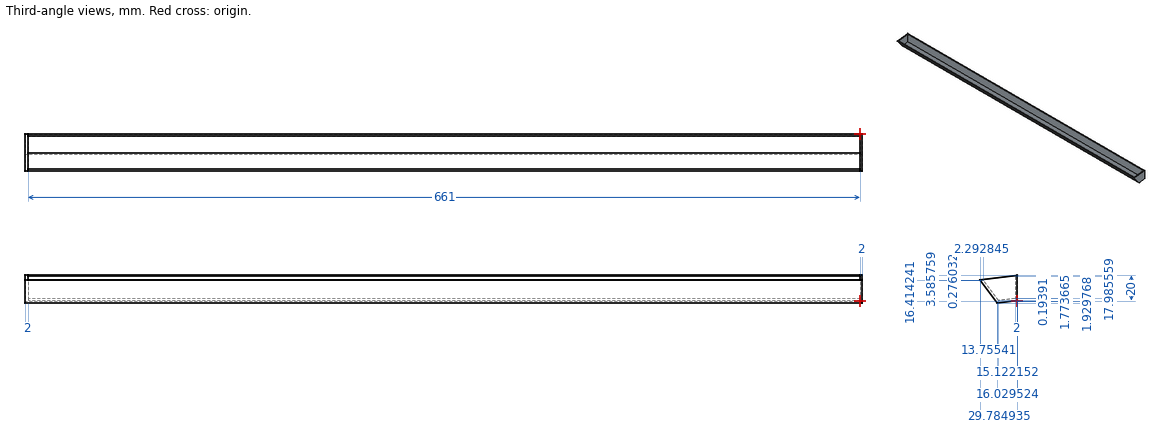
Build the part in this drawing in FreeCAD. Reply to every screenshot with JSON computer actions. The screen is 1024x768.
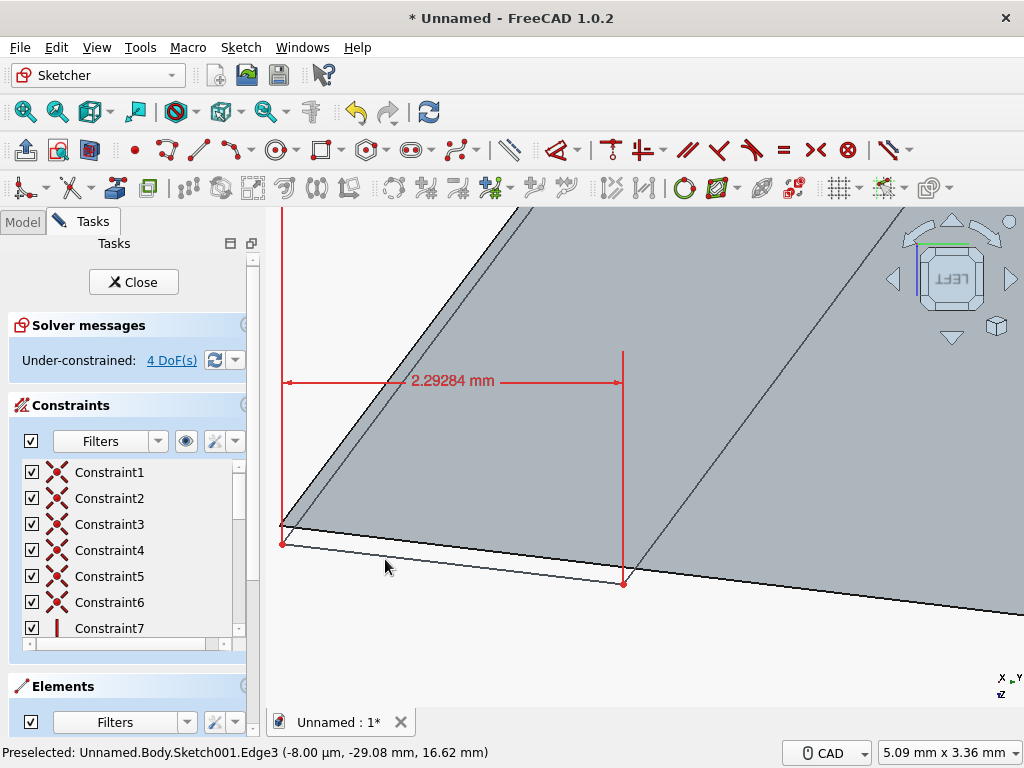
{"action": "left_click", "coordinate": [385, 556]}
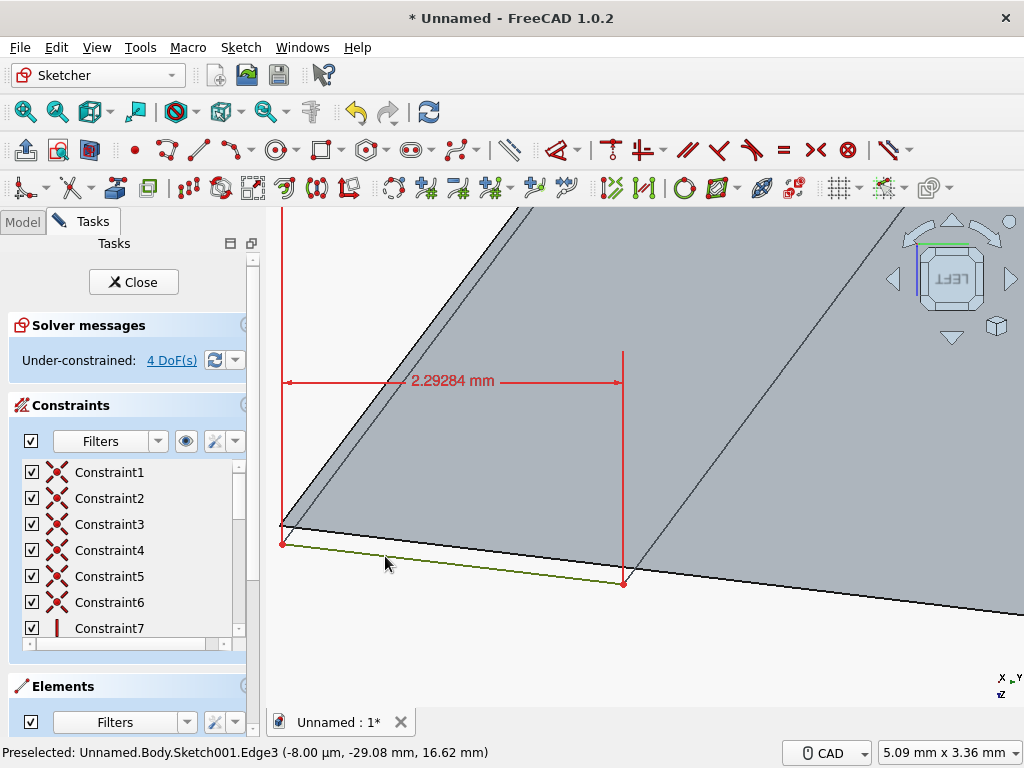
{"action": "left_click", "coordinate": [580, 150]}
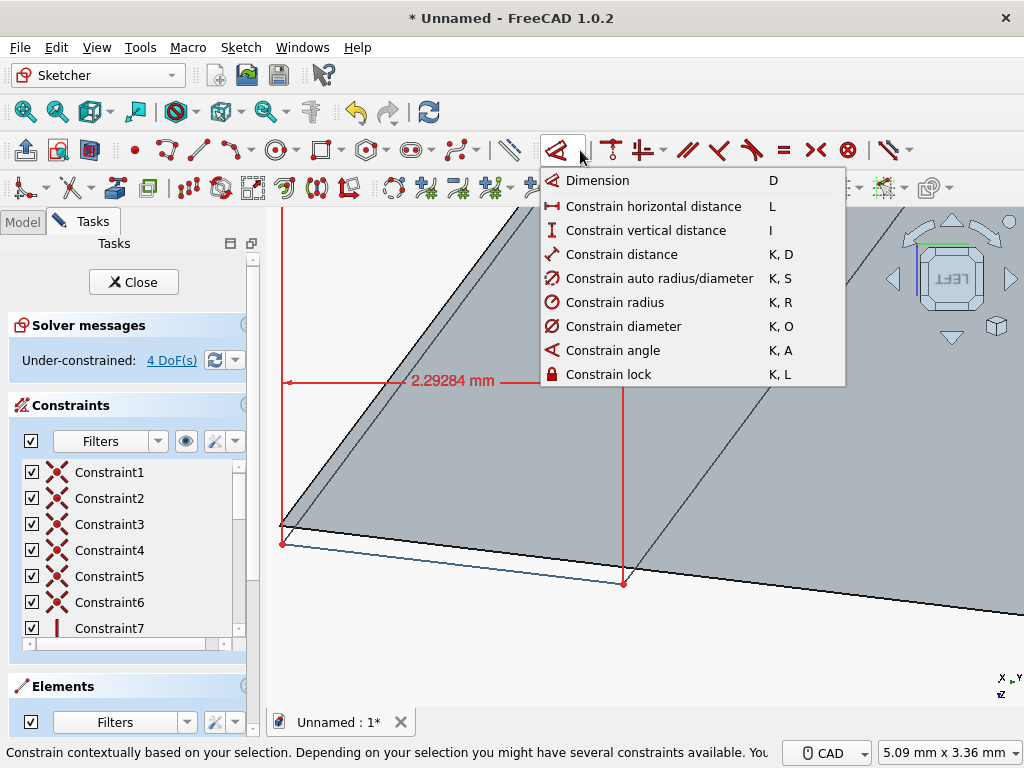
{"action": "left_click", "coordinate": [693, 230]}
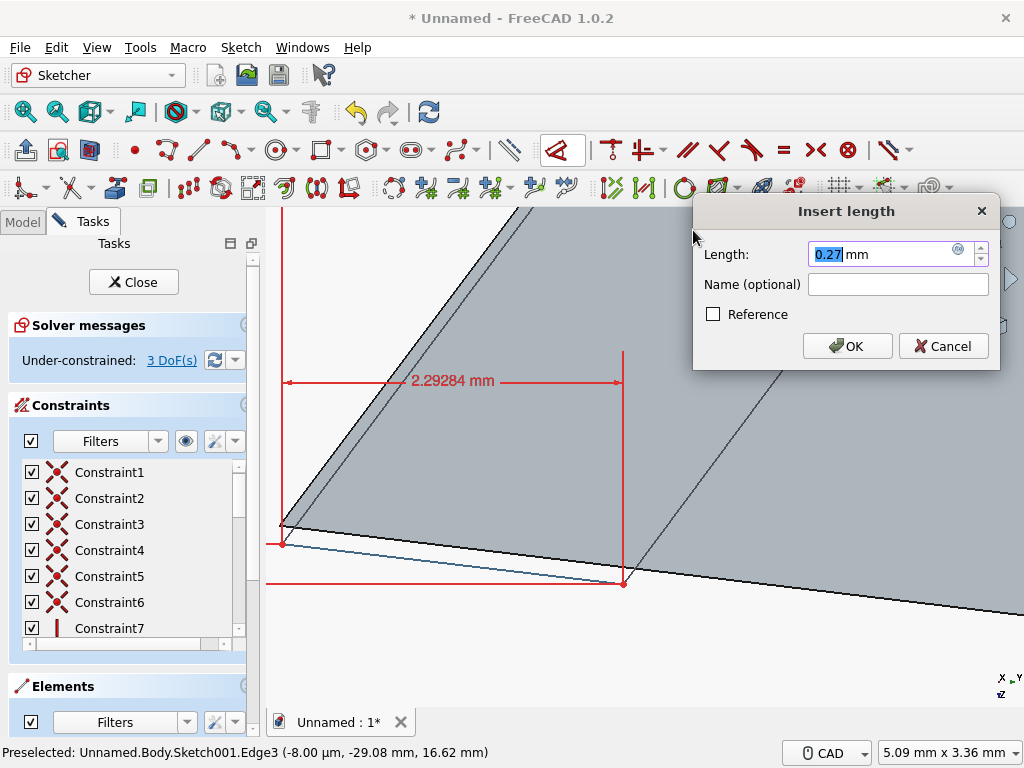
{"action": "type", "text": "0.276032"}
{"action": "key", "text": "Return"}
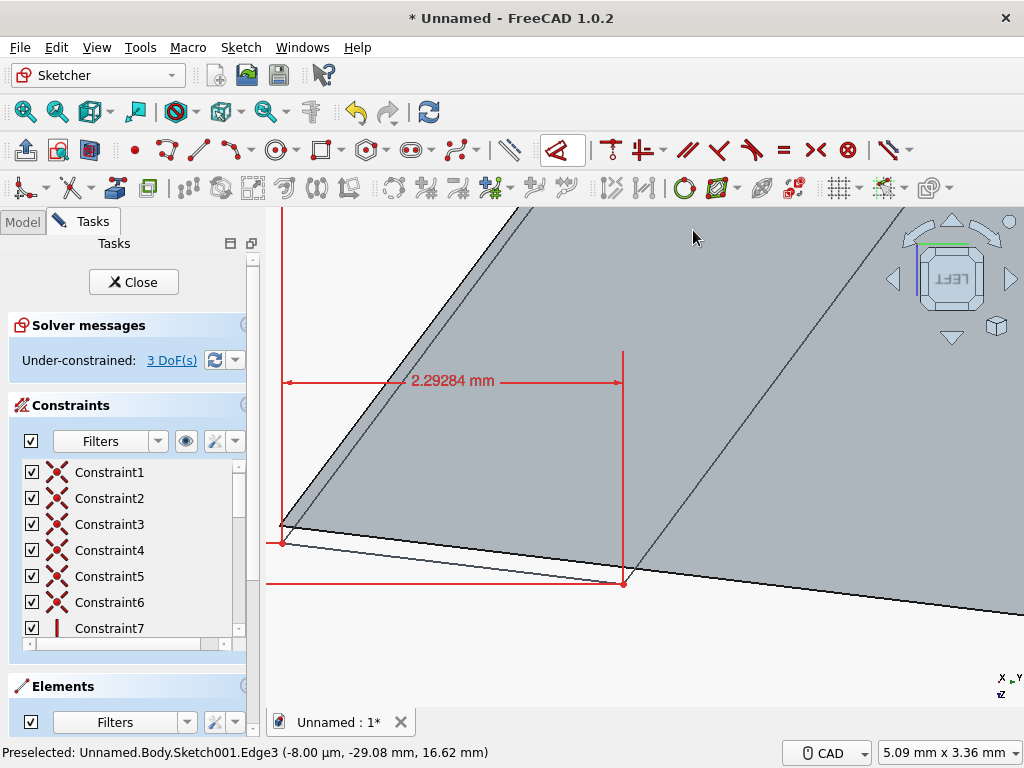
{"action": "scroll", "coordinate": [385, 560], "scroll_direction": "down", "scroll_amount": 12}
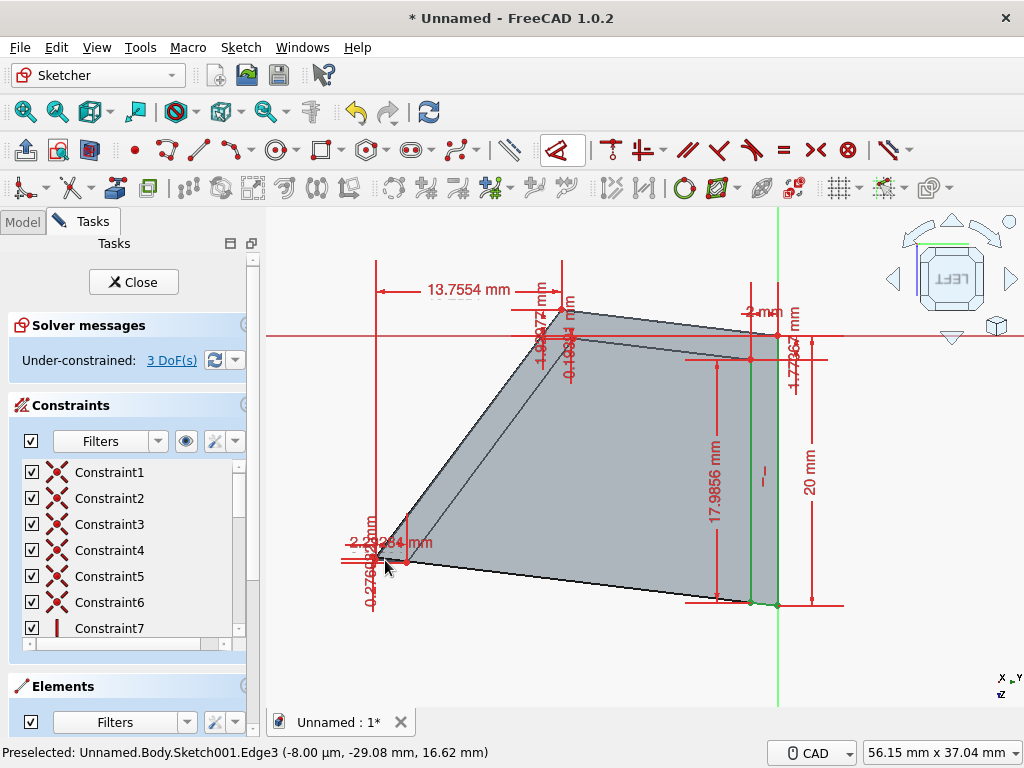
{"action": "left_click", "coordinate": [562, 310]}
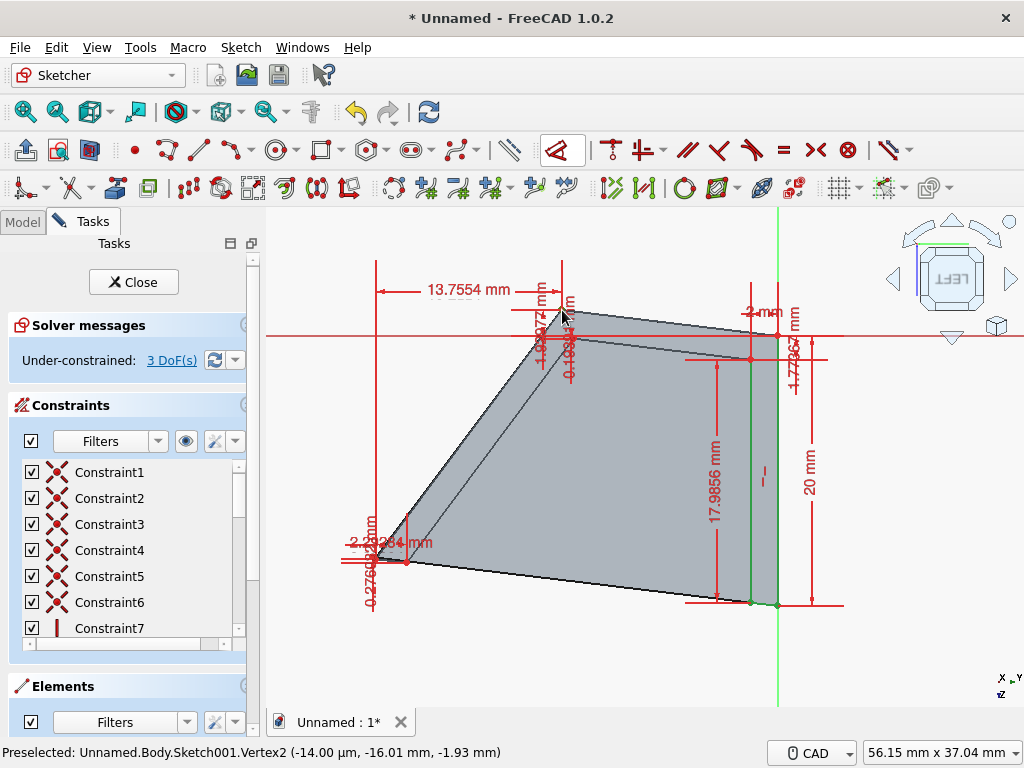
{"action": "key", "text": "l"}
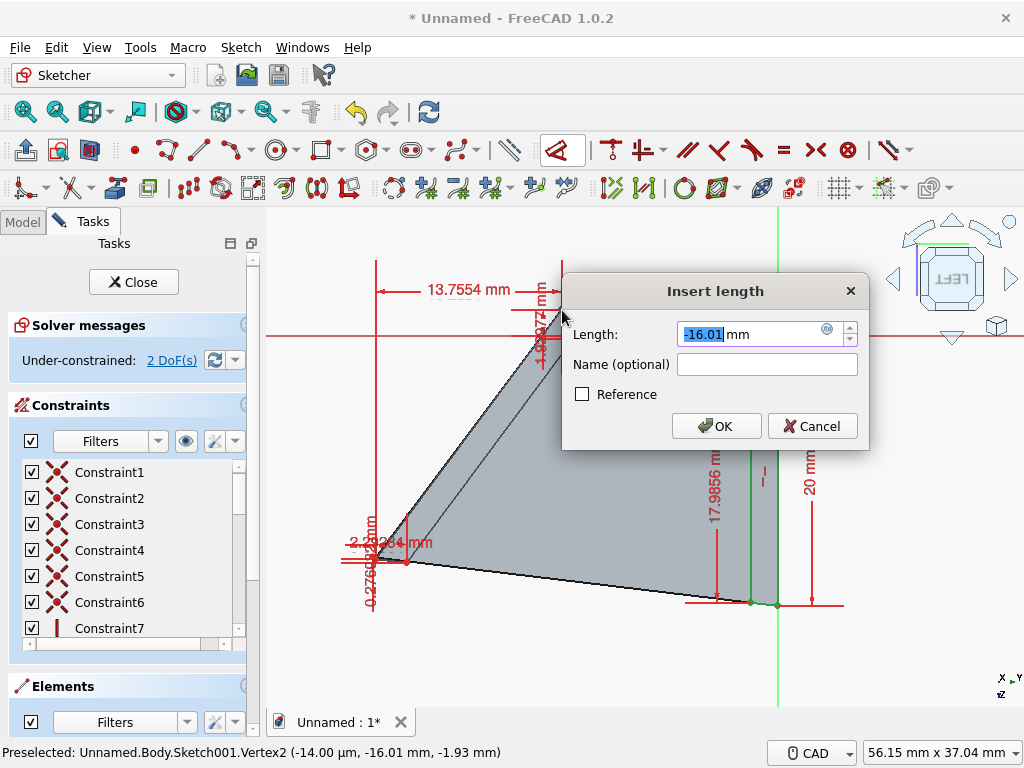
{"action": "type", "text": "-16.029524"}
{"action": "key", "text": "Return"}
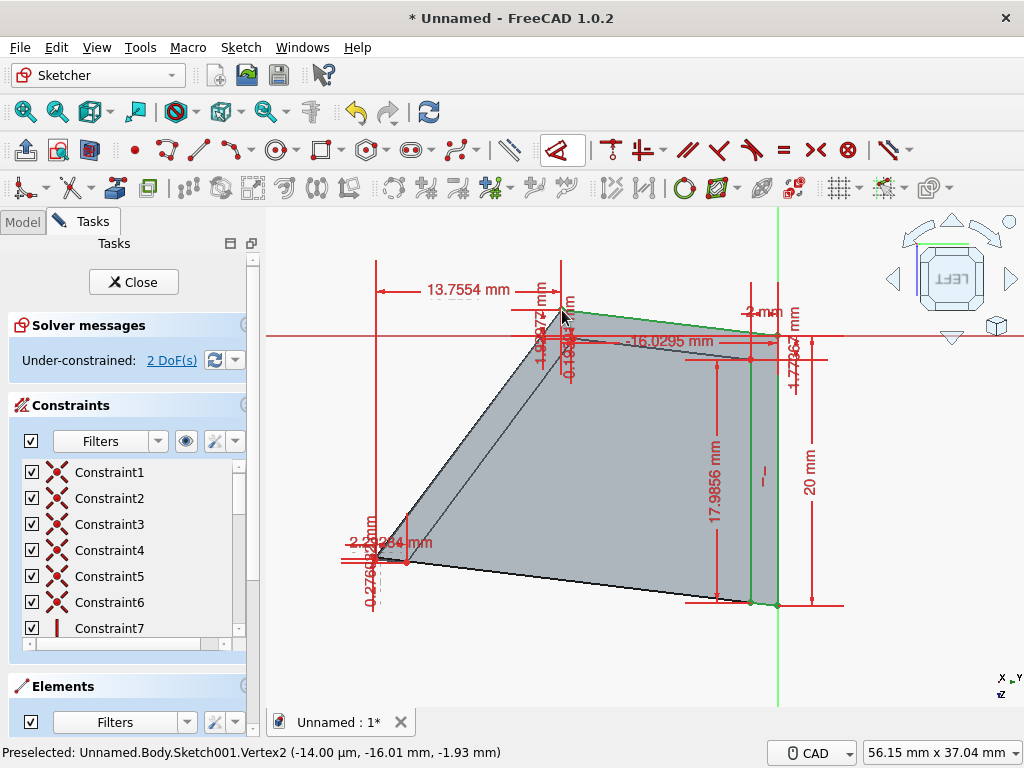
{"action": "left_click", "coordinate": [376, 559]}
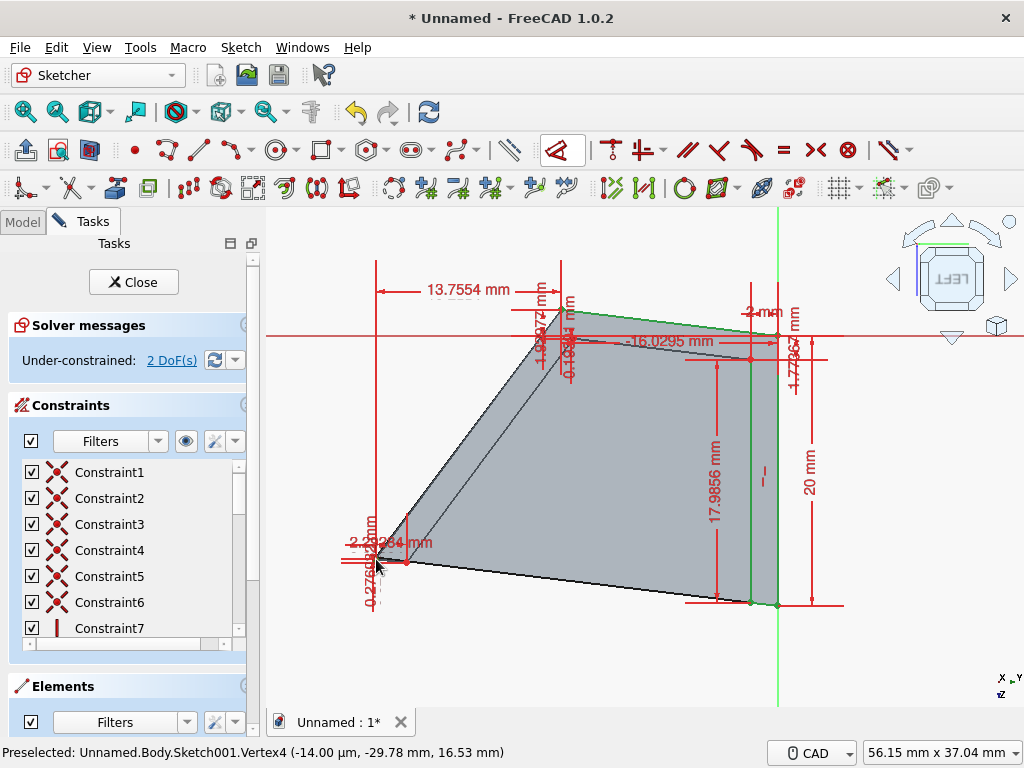
{"action": "left_click", "coordinate": [580, 150]}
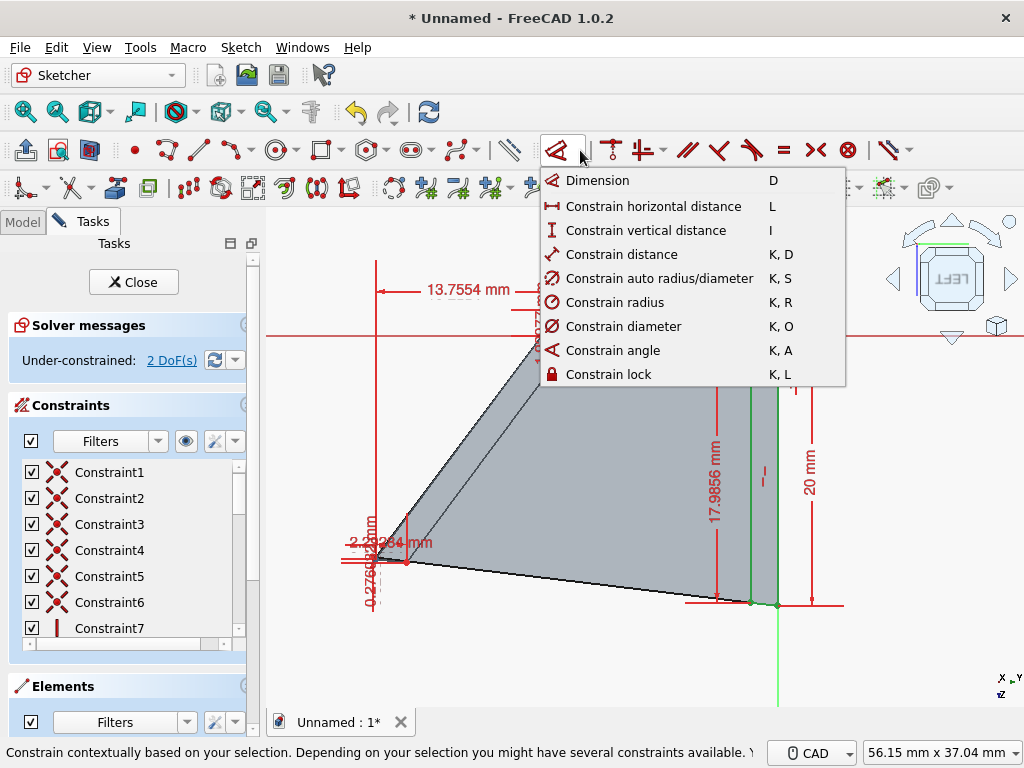
{"action": "left_click", "coordinate": [693, 230]}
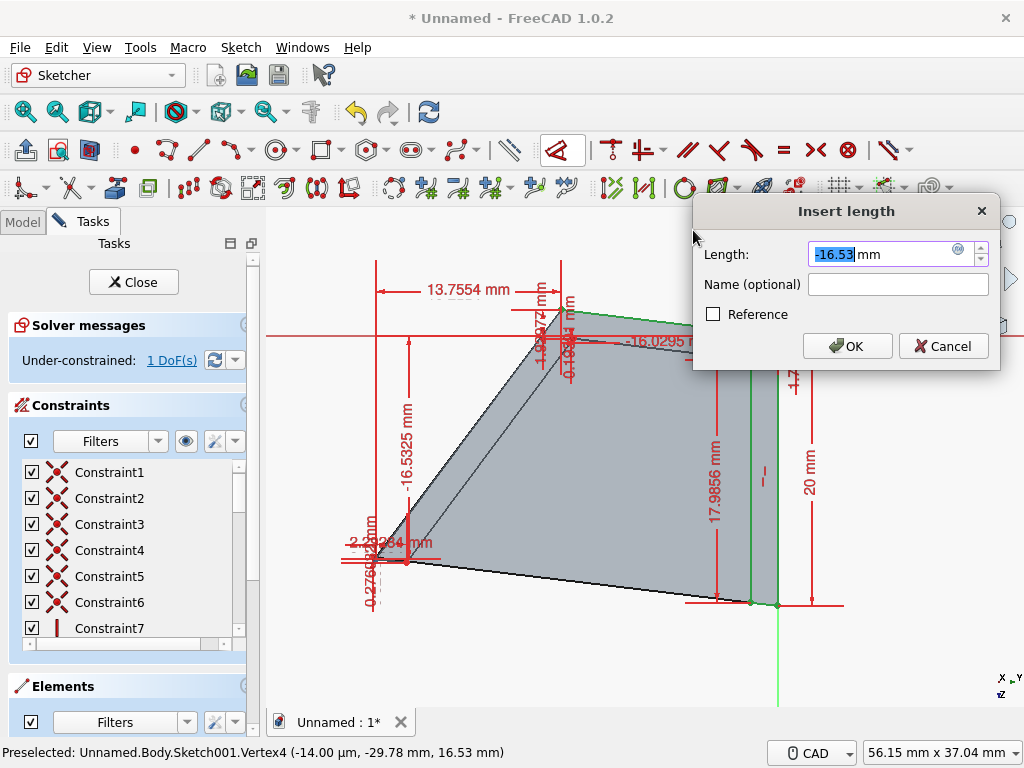
{"action": "type", "text": "-16.414241"}
{"action": "key", "text": "Return"}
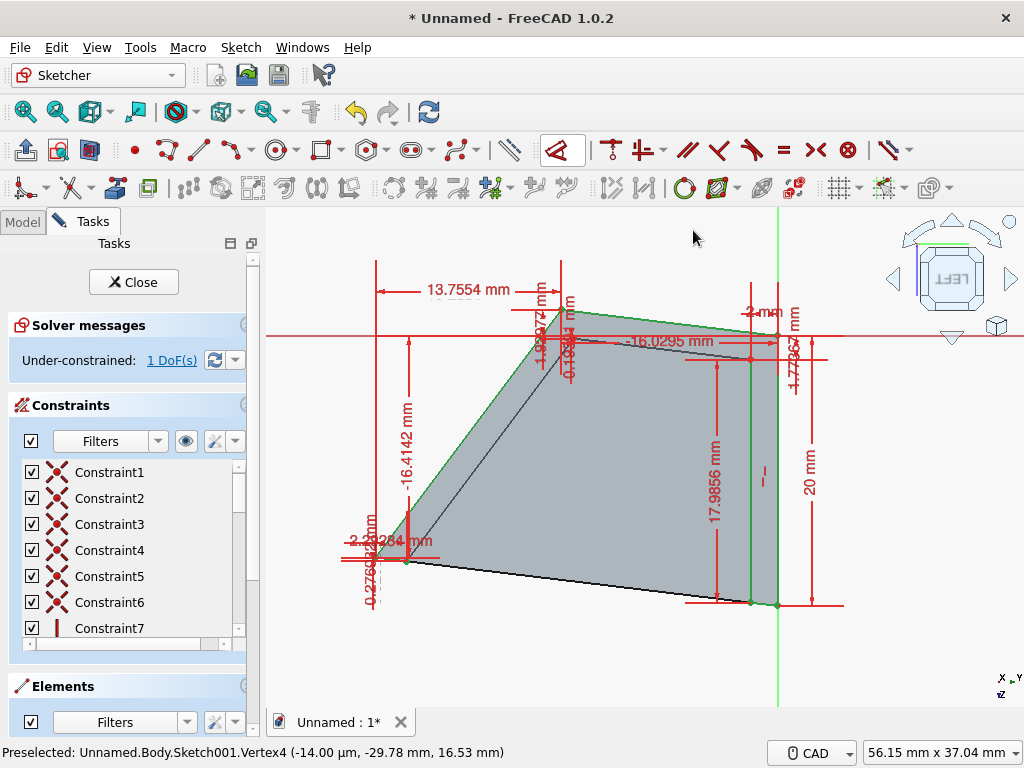
{"action": "left_click", "coordinate": [573, 339]}